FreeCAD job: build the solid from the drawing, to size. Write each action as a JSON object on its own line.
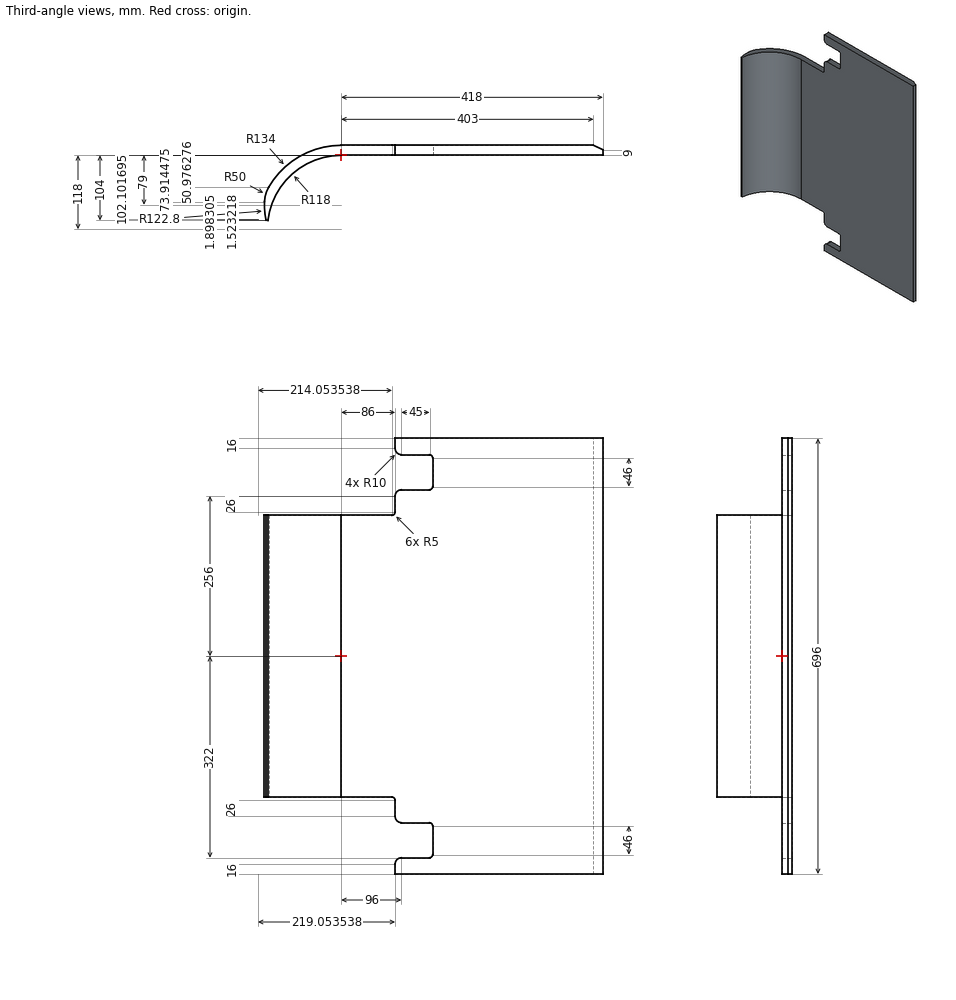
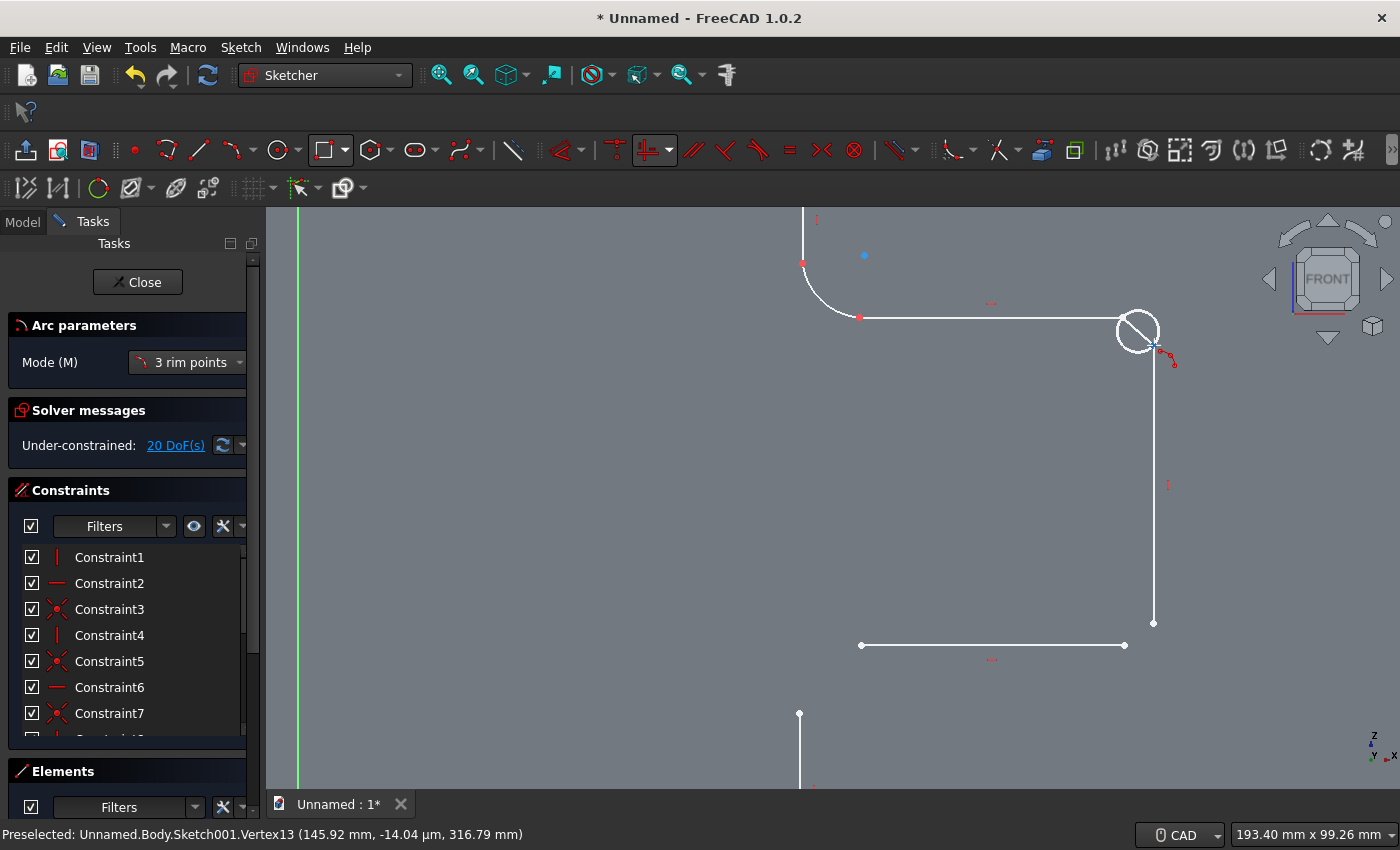
{"action": "scroll", "coordinate": [1146, 323], "scroll_direction": "up", "scroll_amount": 4}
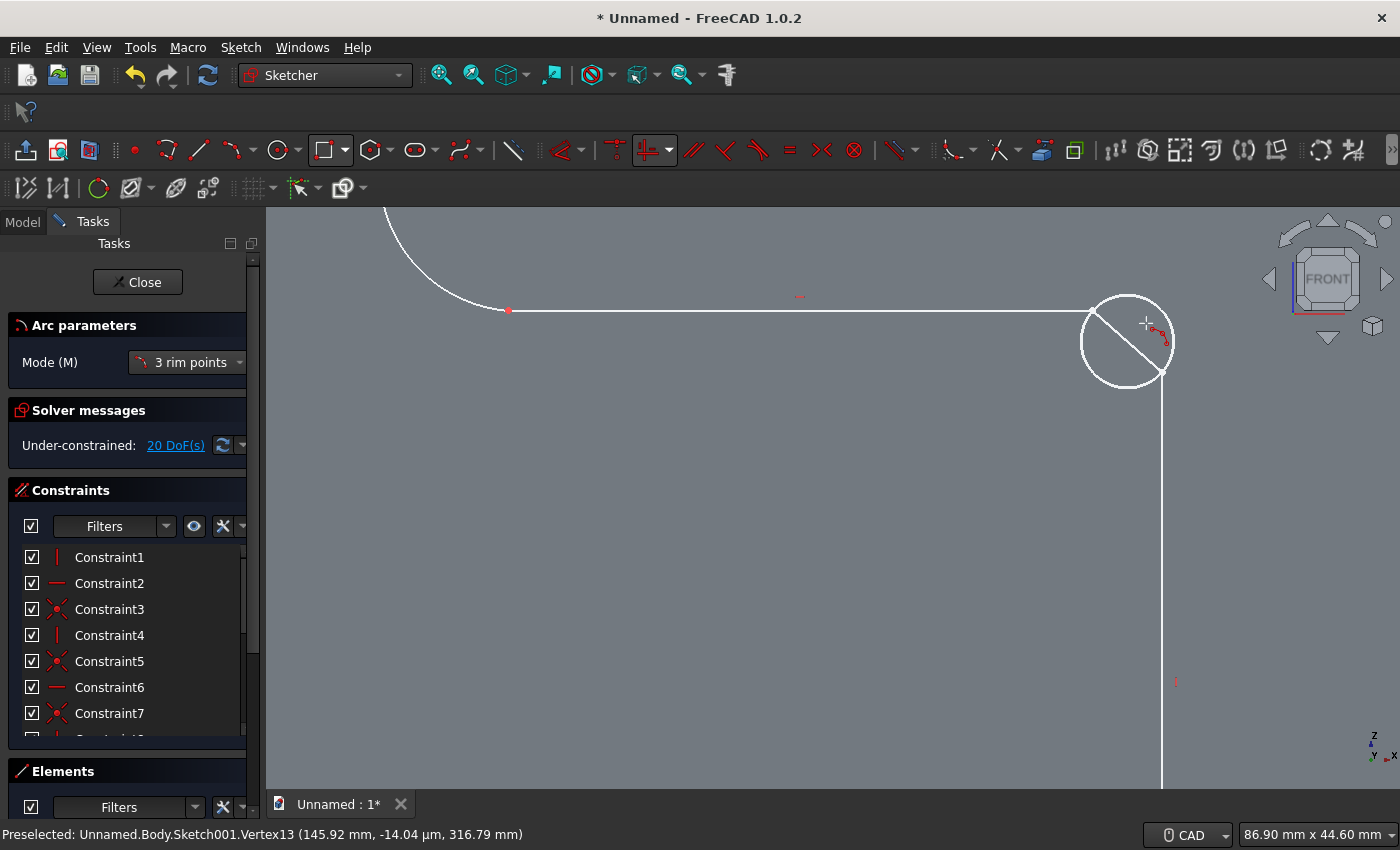
{"action": "left_click", "coordinate": [1144, 323]}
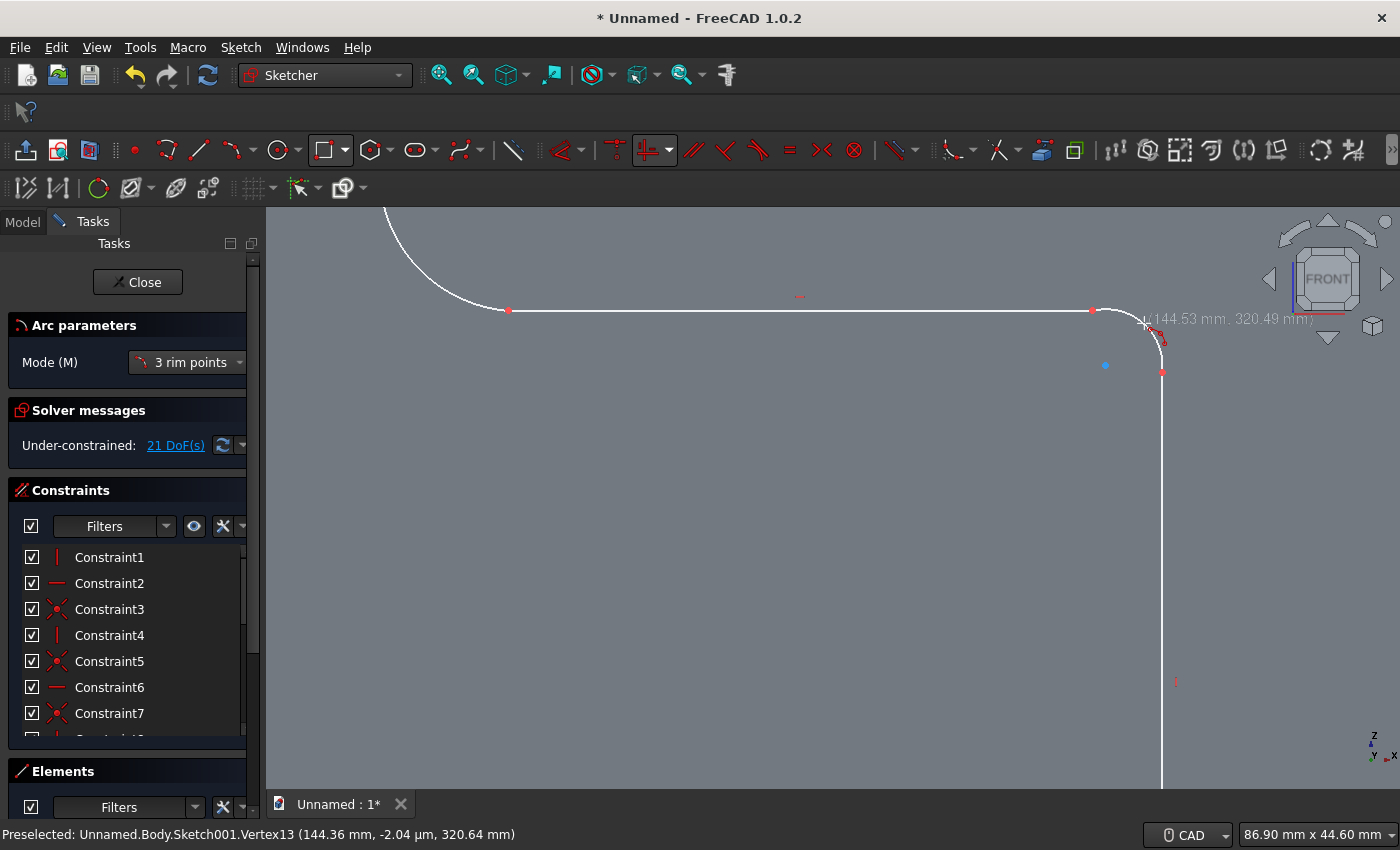
{"action": "scroll", "coordinate": [839, 288], "scroll_direction": "down", "scroll_amount": 15}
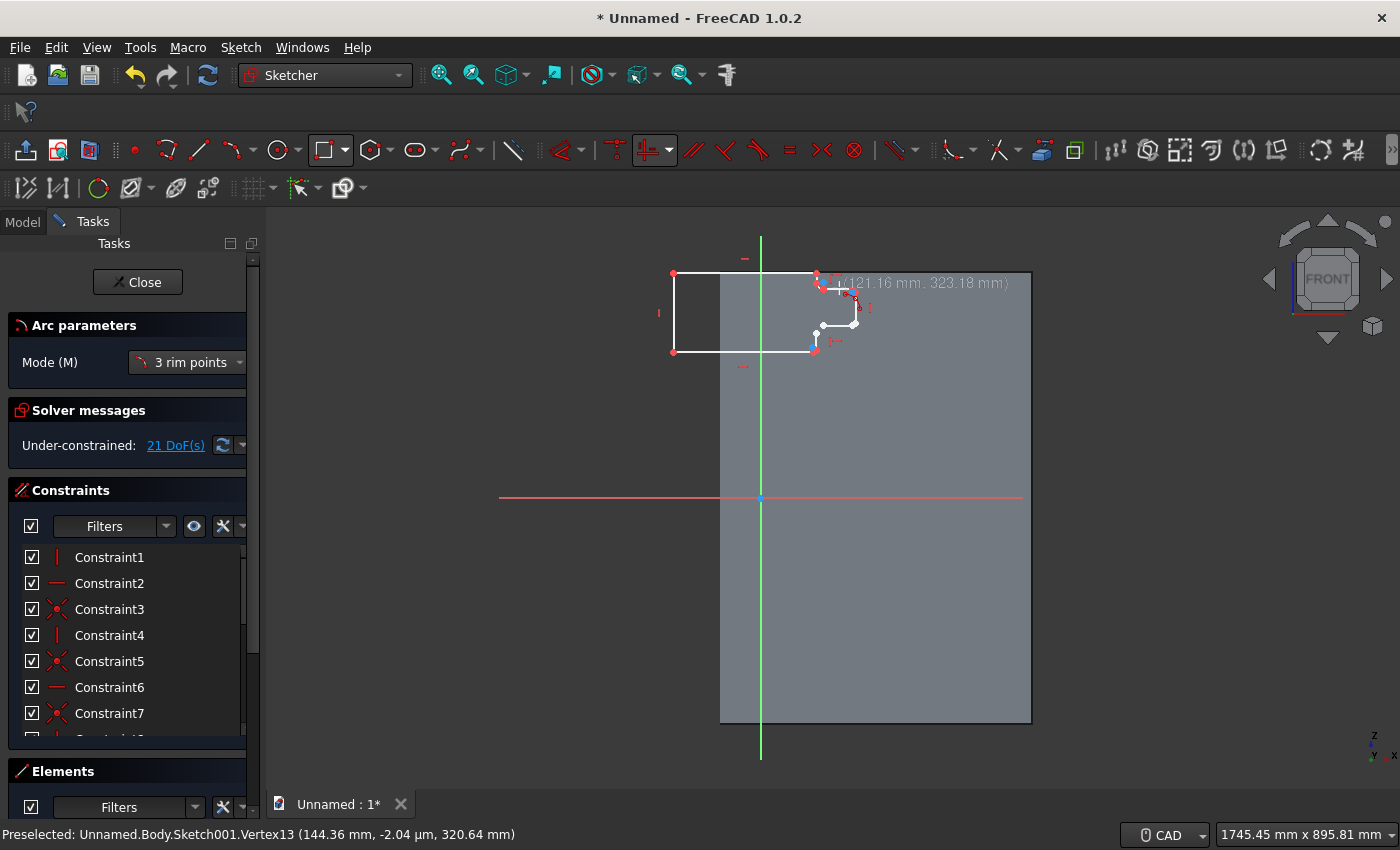
{"action": "scroll", "coordinate": [856, 322], "scroll_direction": "up", "scroll_amount": 7}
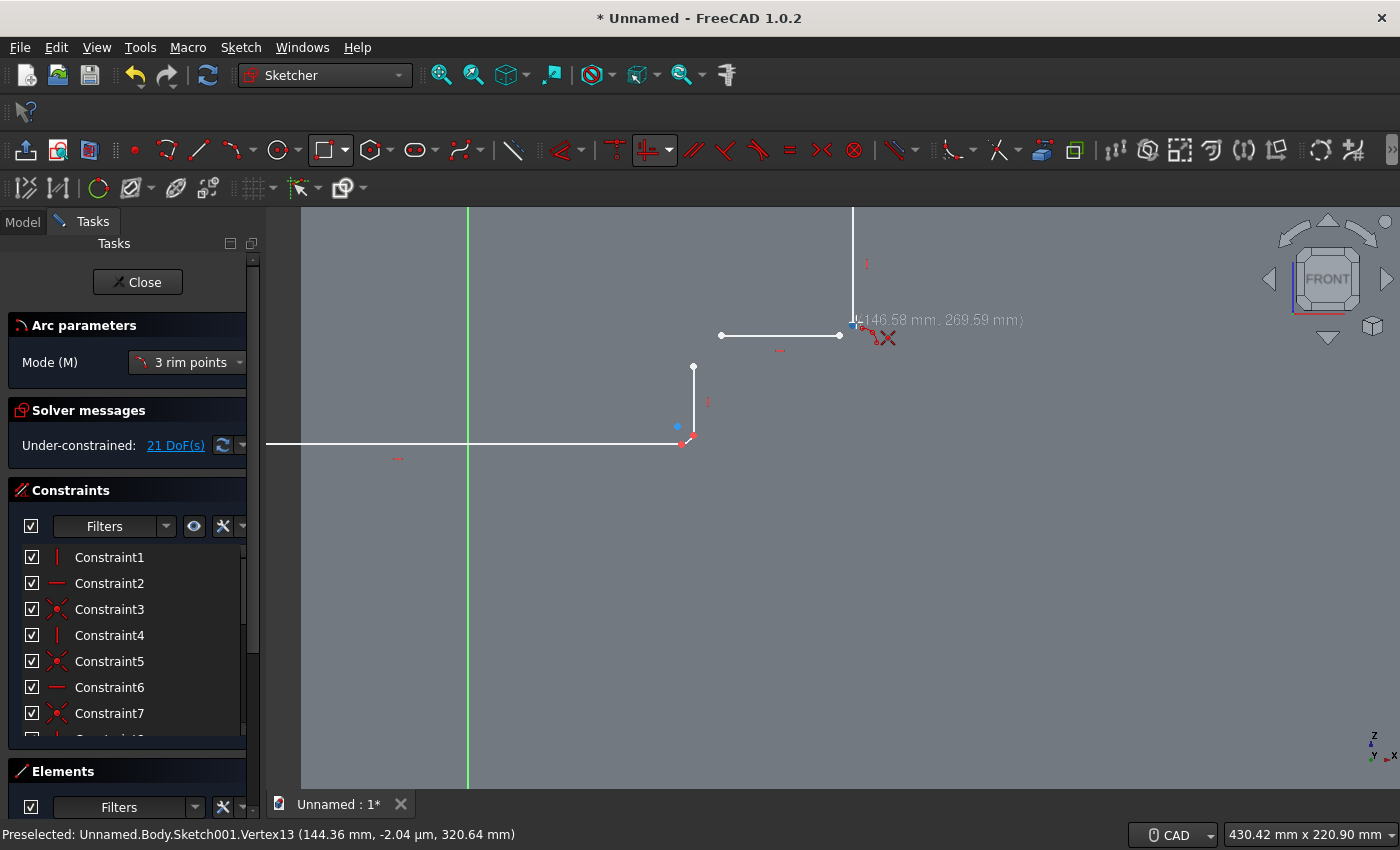
{"action": "left_click", "coordinate": [853, 326]}
{"action": "left_click", "coordinate": [839, 336]}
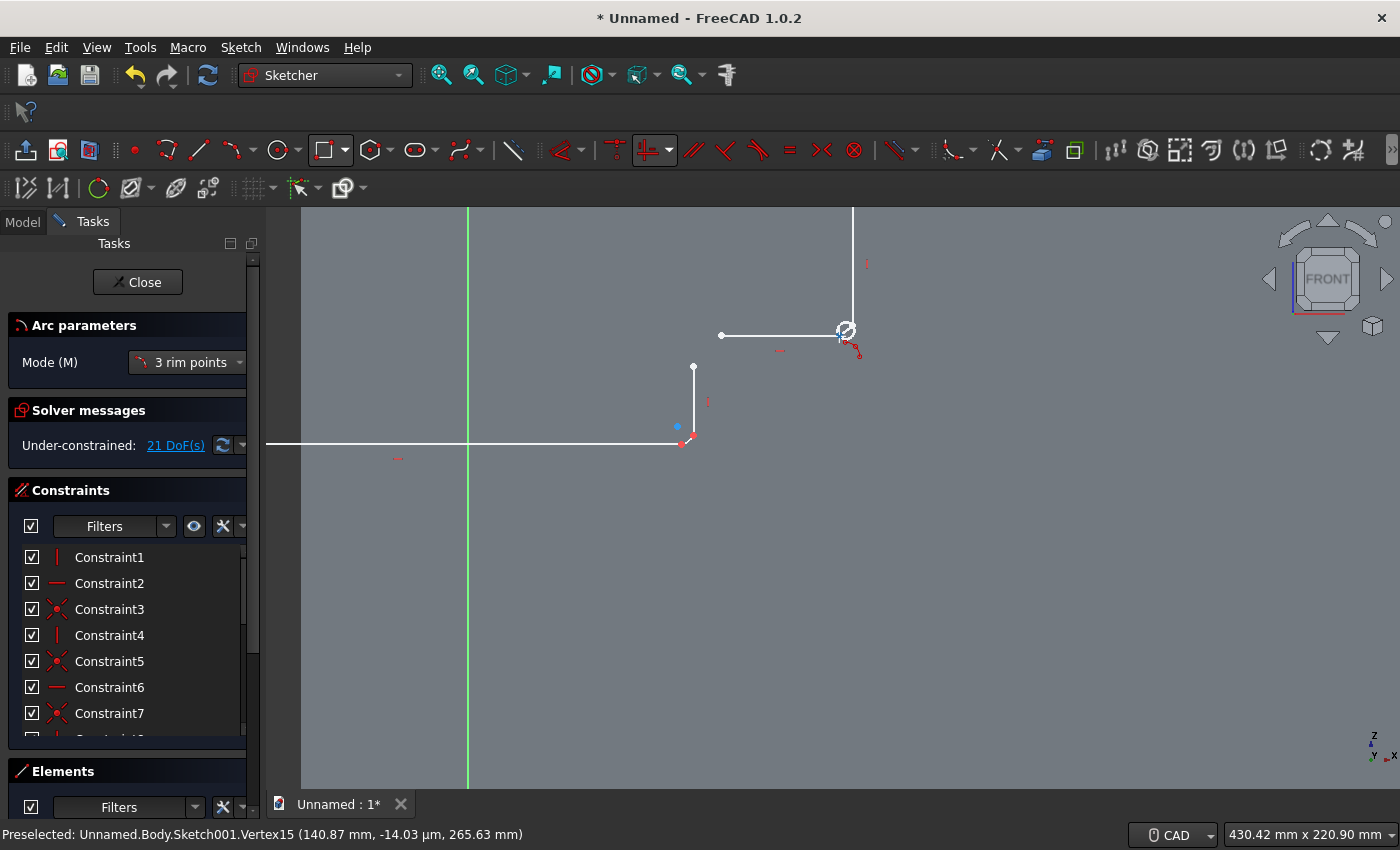
{"action": "scroll", "coordinate": [849, 331], "scroll_direction": "up", "scroll_amount": 8}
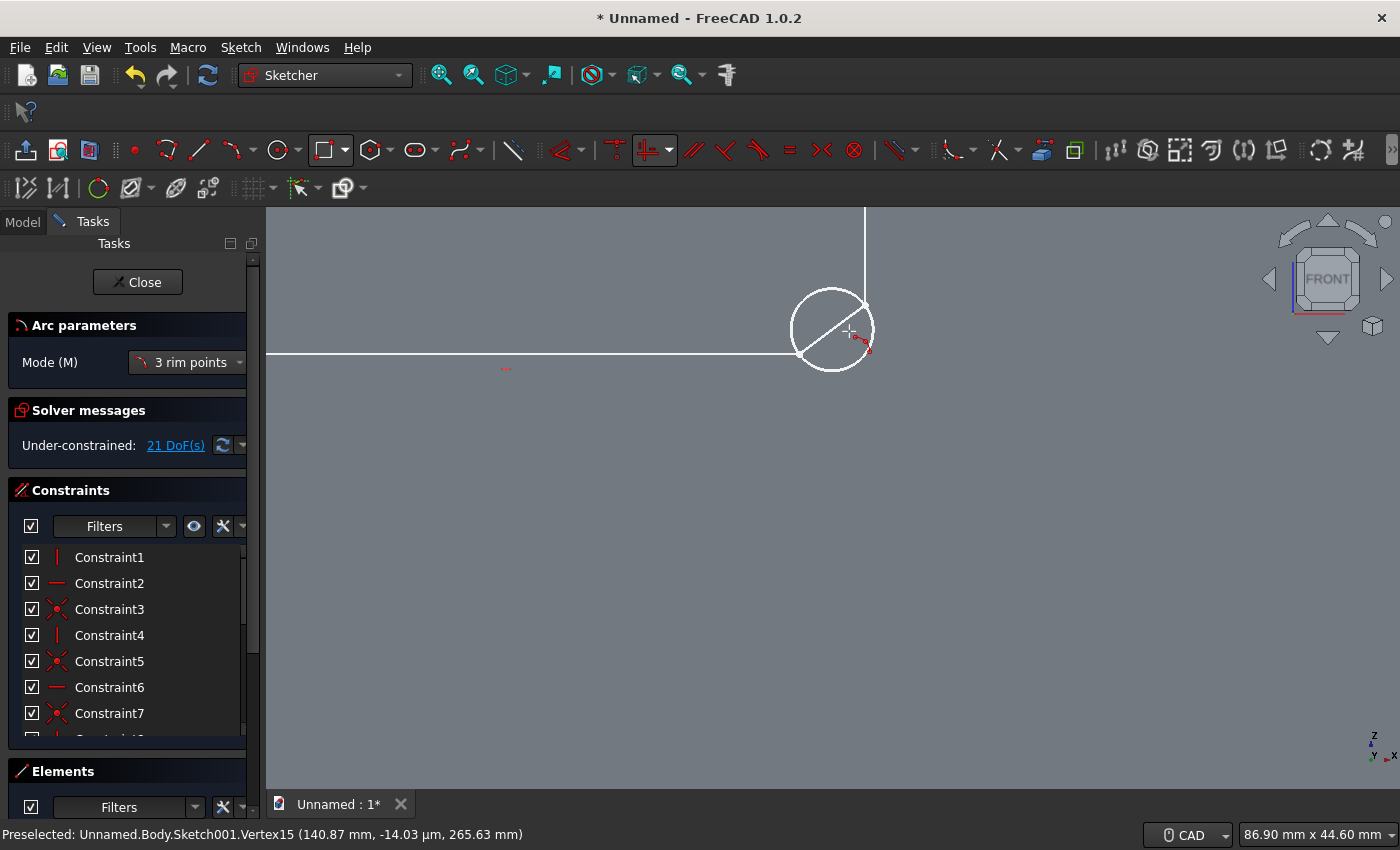
{"action": "left_click", "coordinate": [847, 330]}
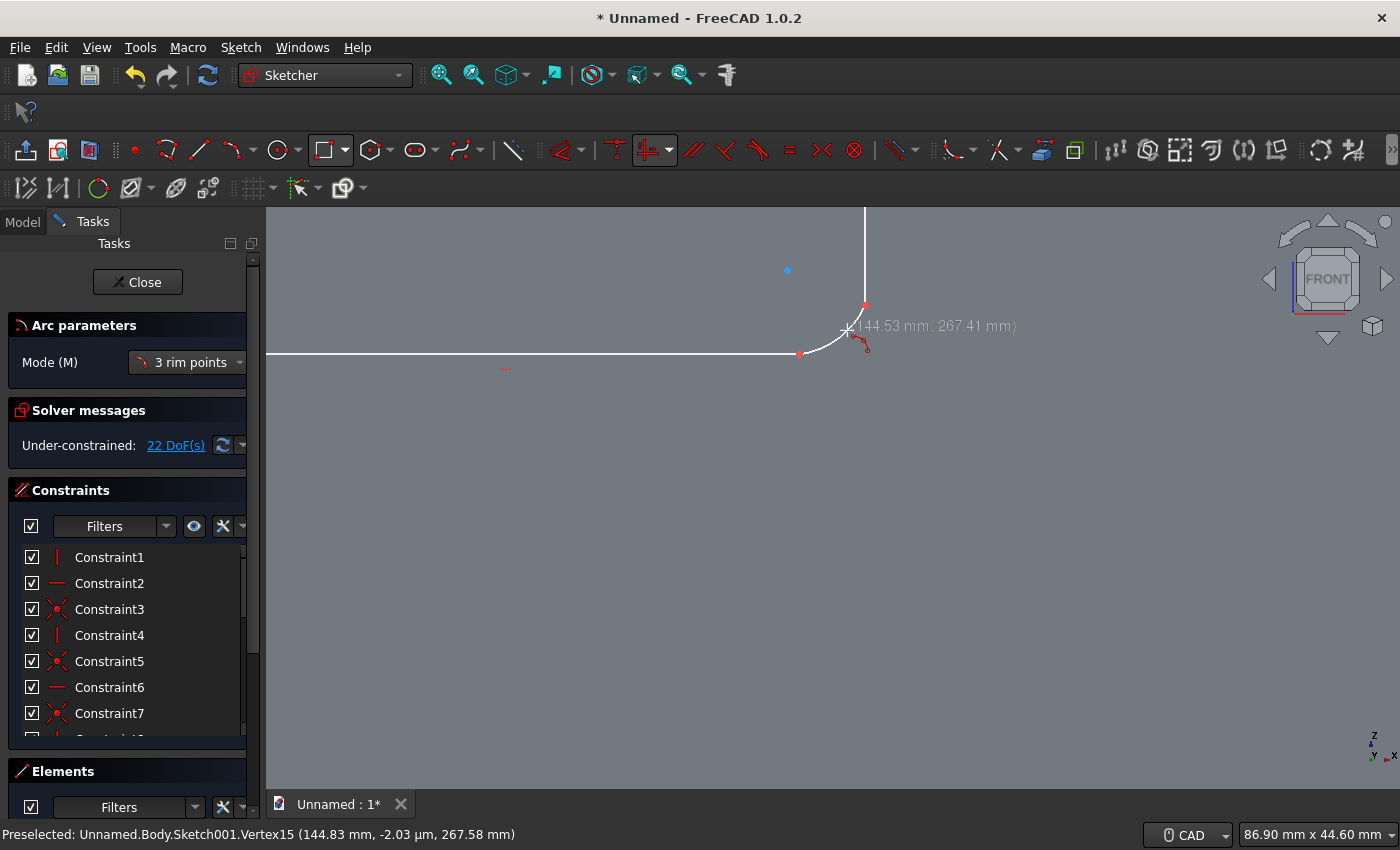
{"action": "scroll", "coordinate": [855, 324], "scroll_direction": "down", "scroll_amount": 15}